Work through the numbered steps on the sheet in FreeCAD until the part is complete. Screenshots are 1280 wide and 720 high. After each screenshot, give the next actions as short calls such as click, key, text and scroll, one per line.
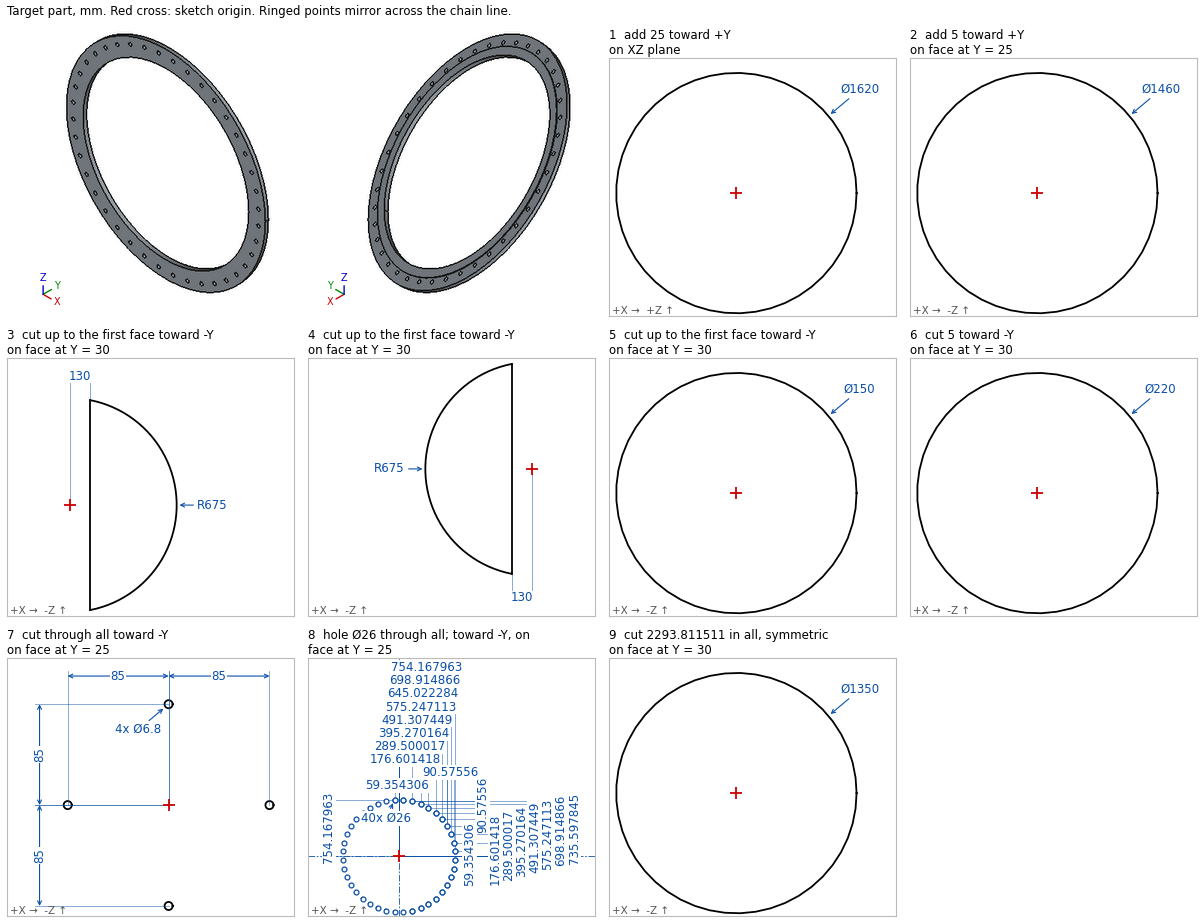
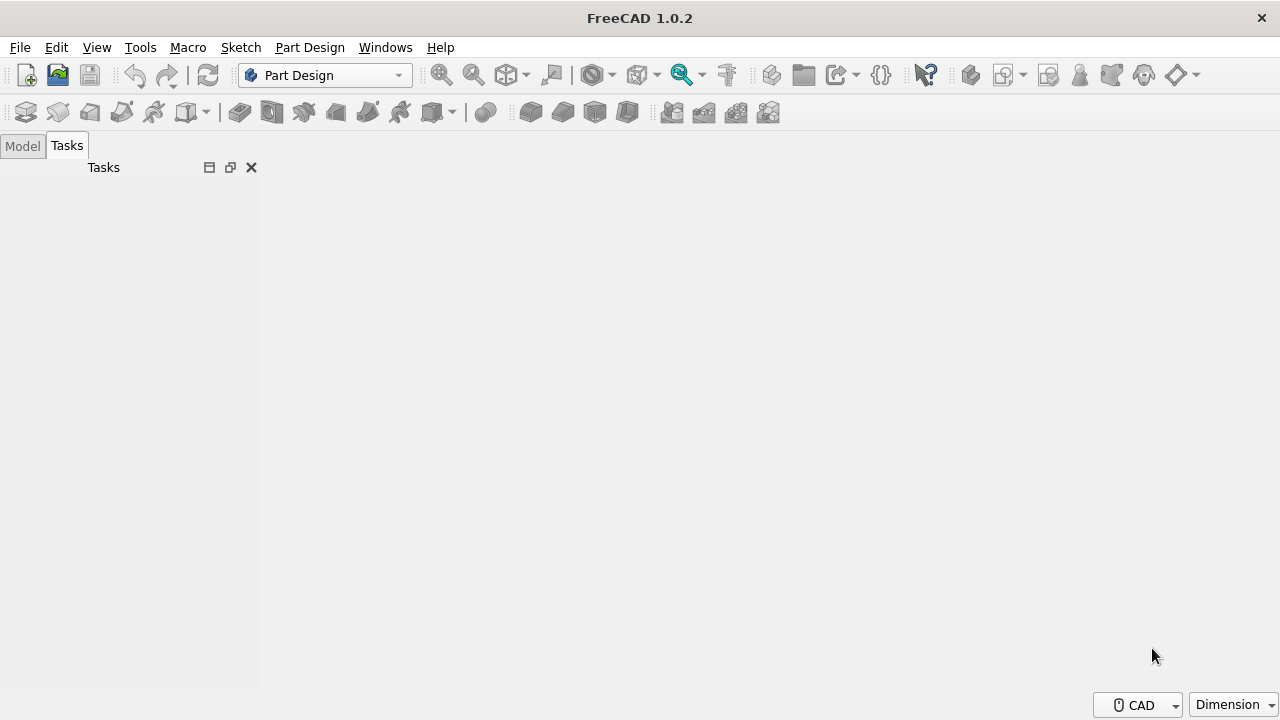
key(ctrl+n)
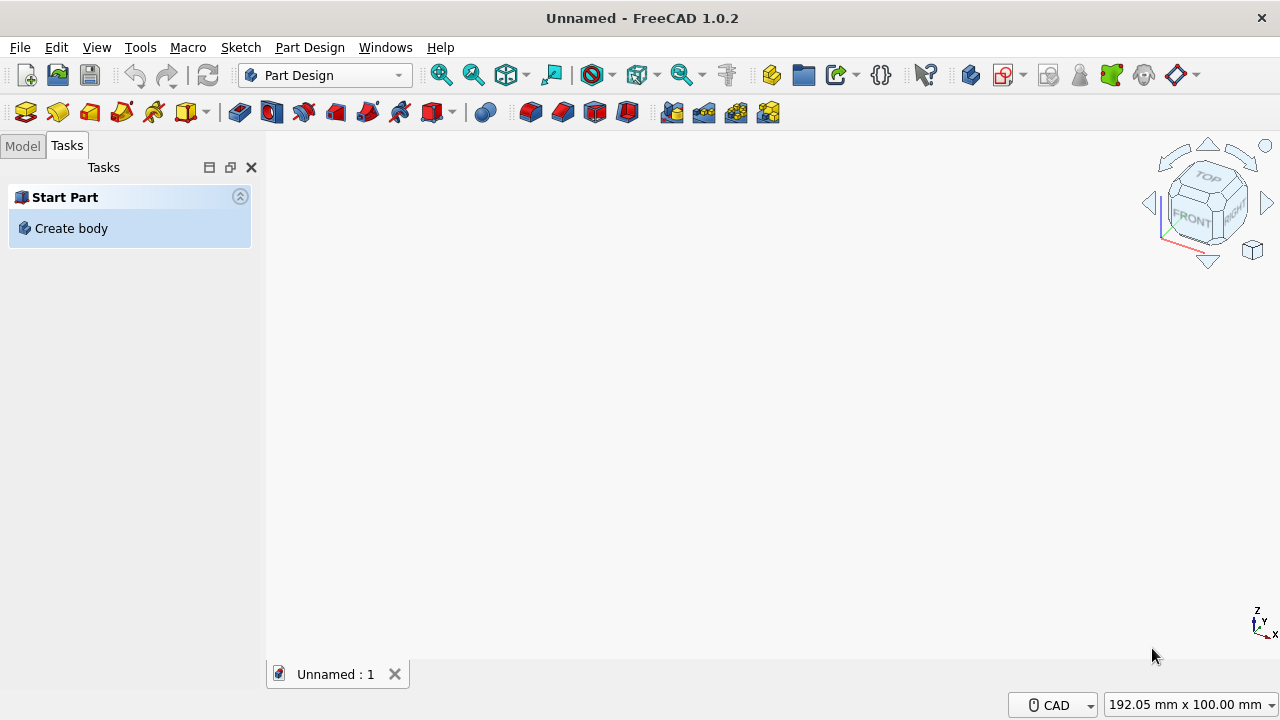
click(1004, 76)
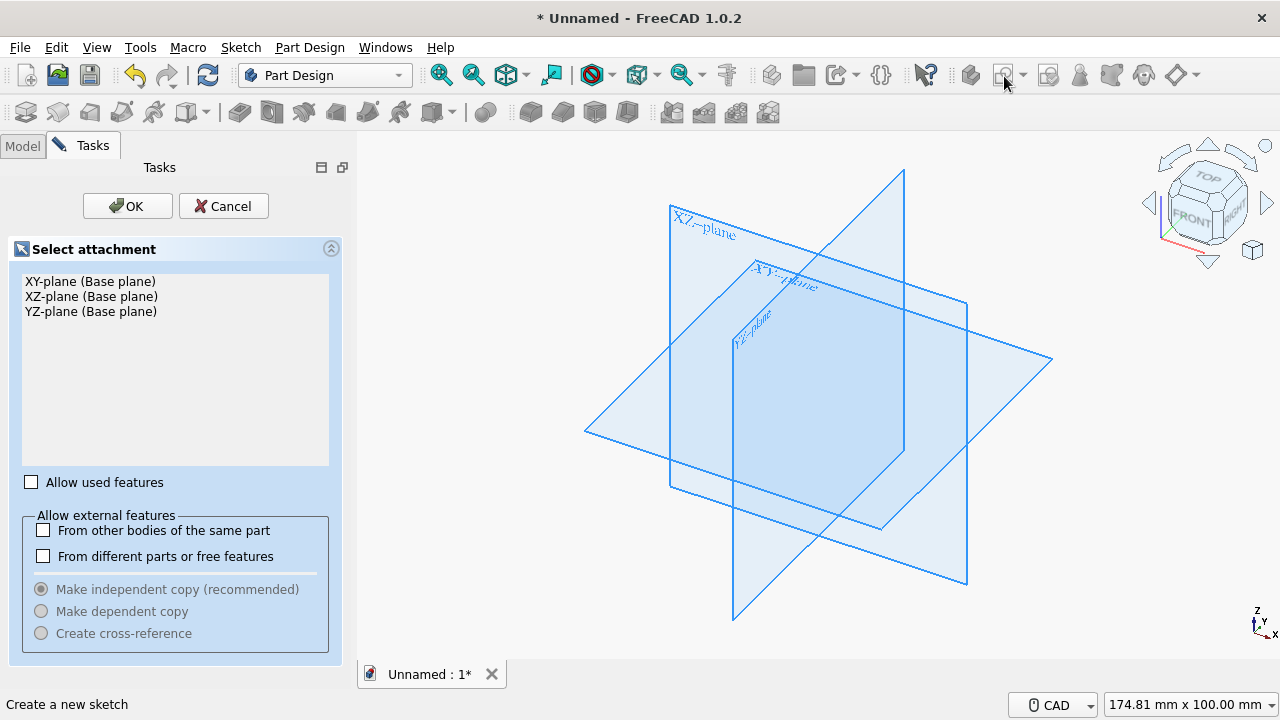
click(82, 296)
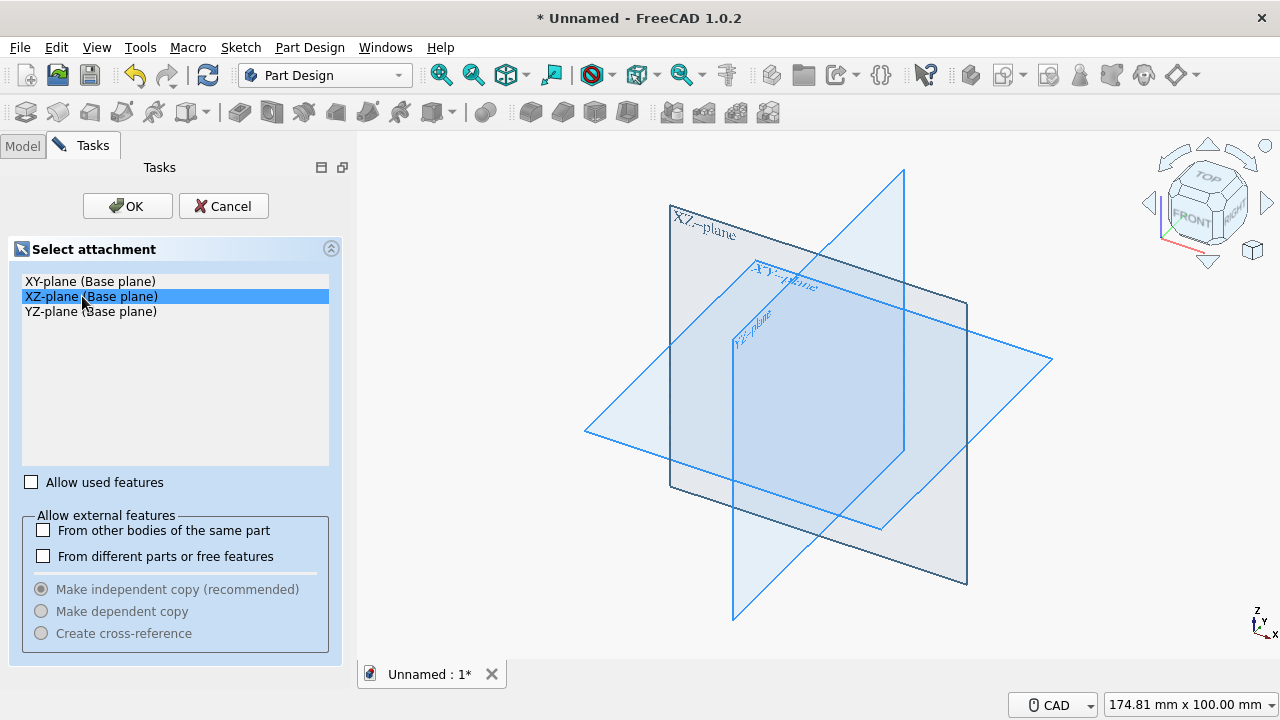
click(128, 206)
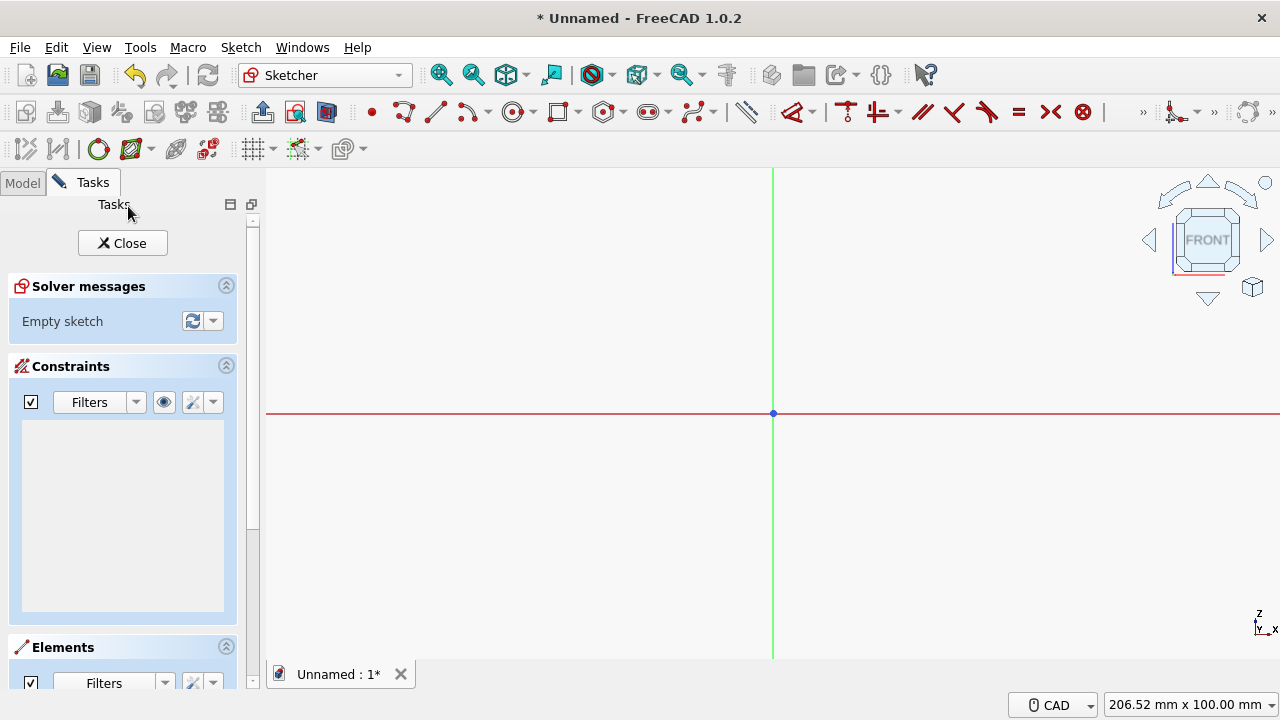
scroll(702, 414, down, 16)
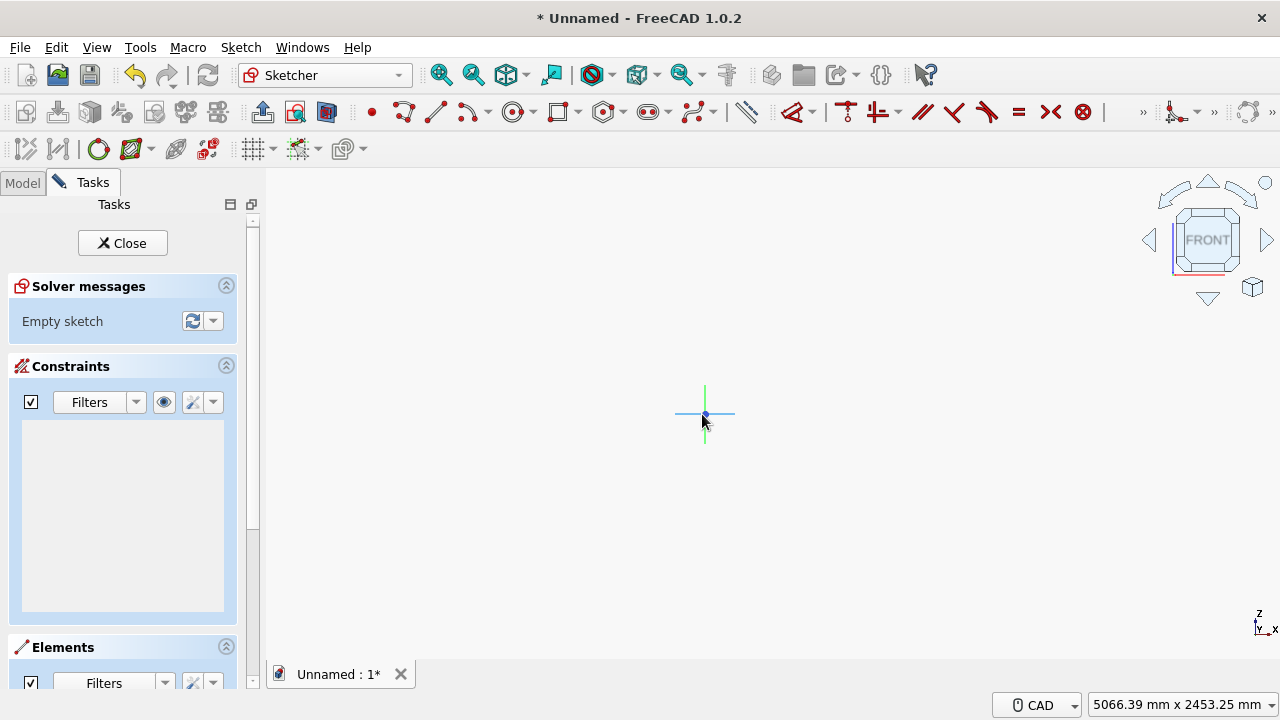
click(514, 112)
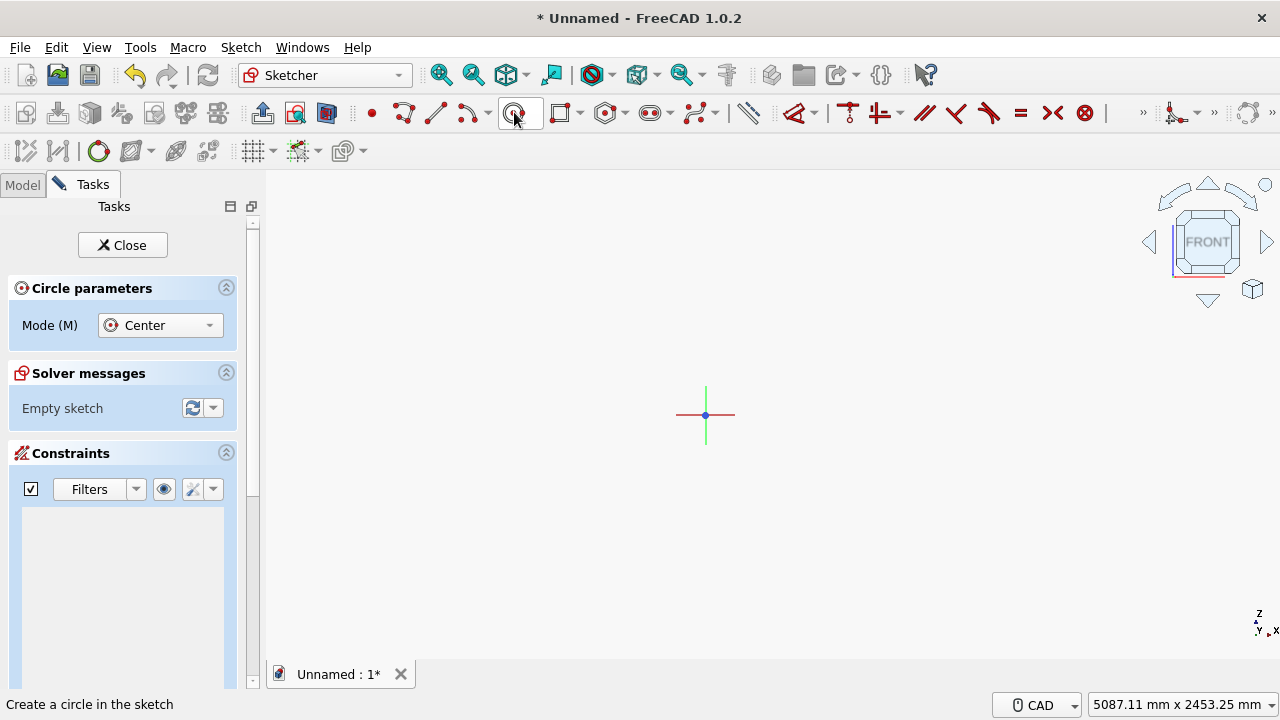
click(706, 415)
click(820, 301)
key(Escape)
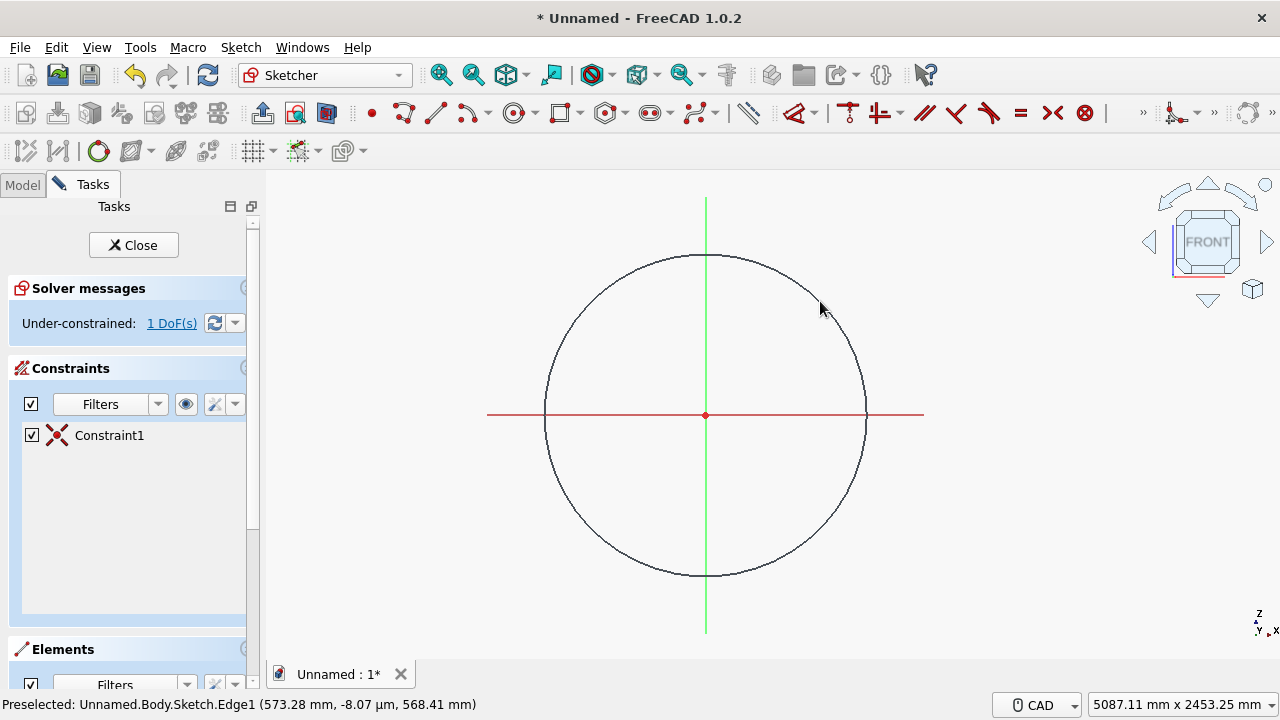
click(819, 301)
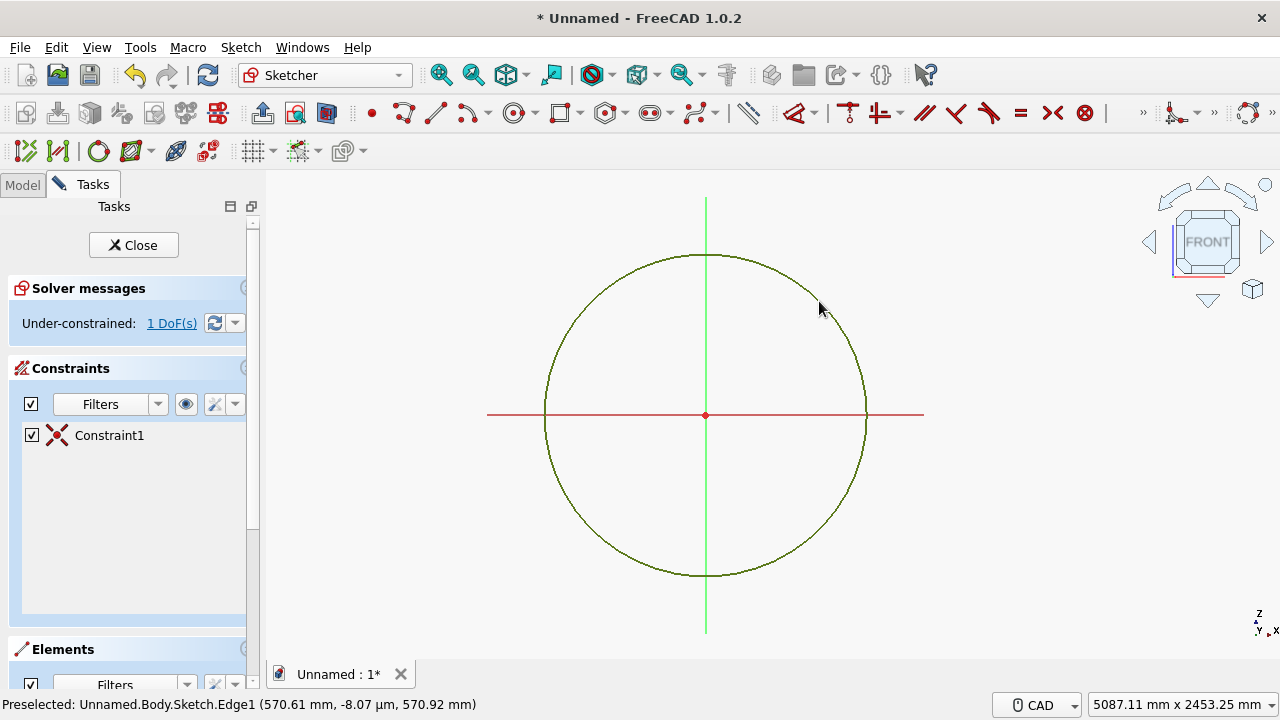
click(816, 114)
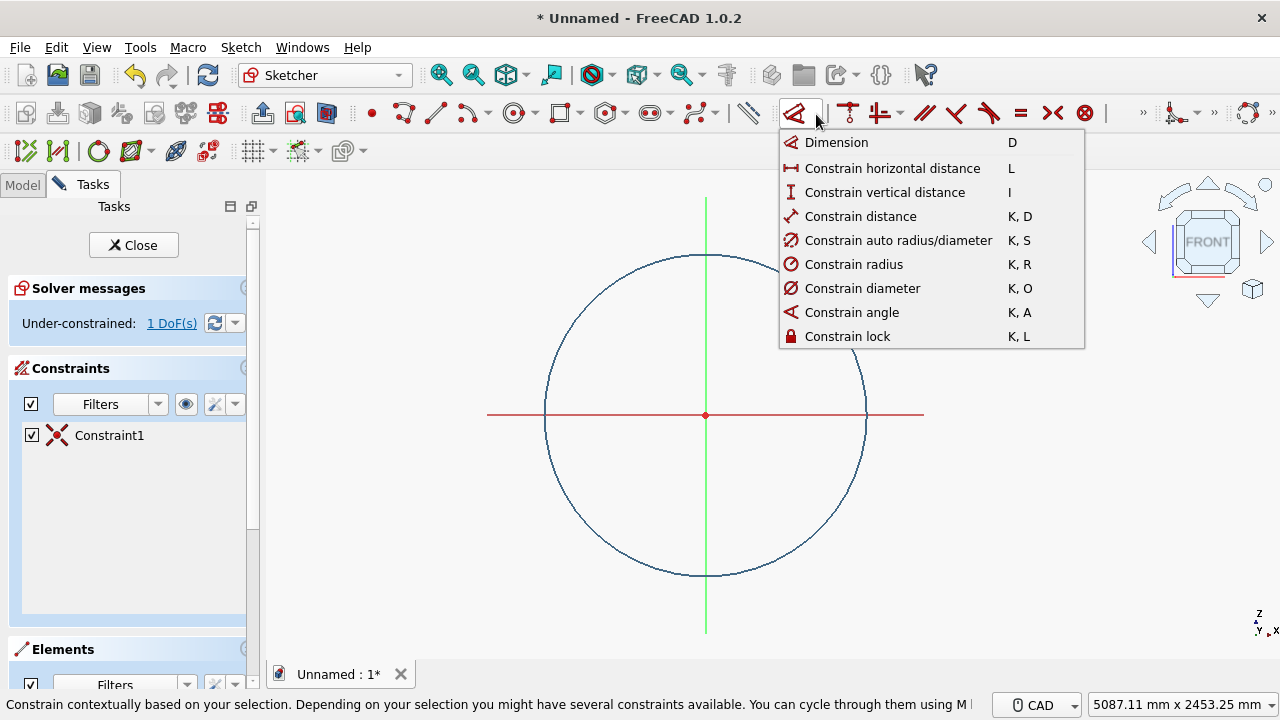
click(932, 288)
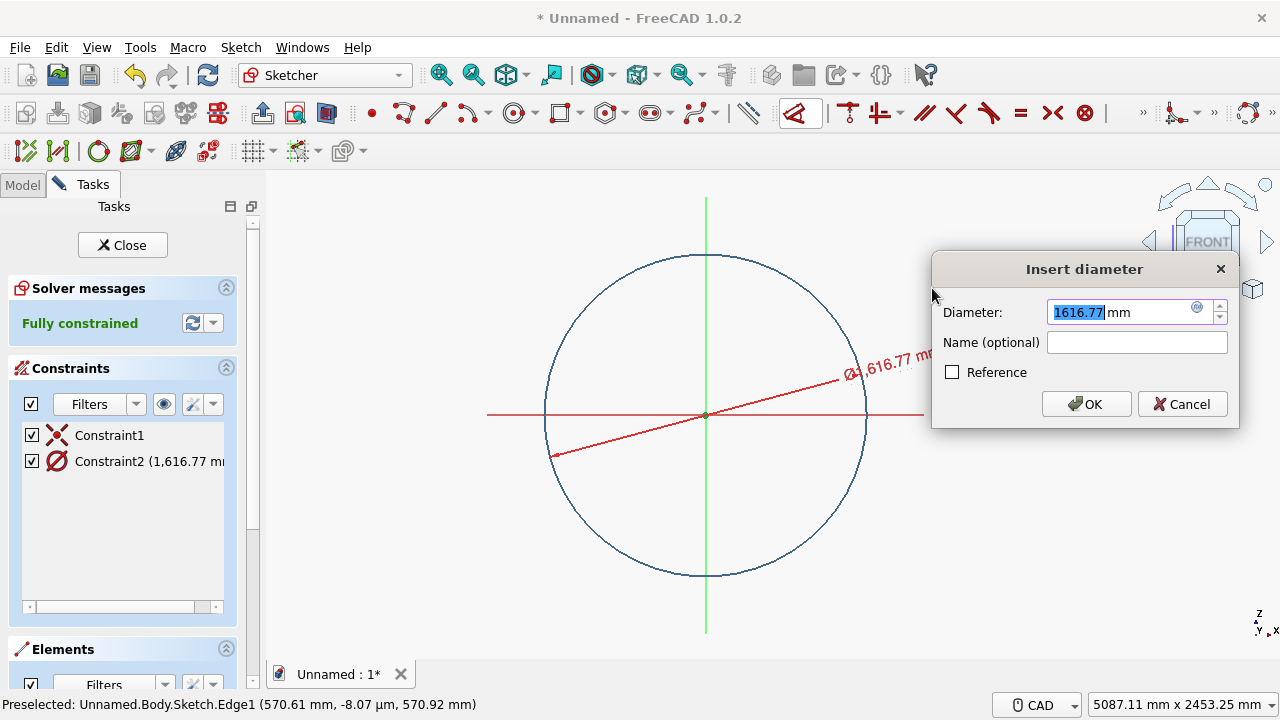
text(1620)
key(Return)